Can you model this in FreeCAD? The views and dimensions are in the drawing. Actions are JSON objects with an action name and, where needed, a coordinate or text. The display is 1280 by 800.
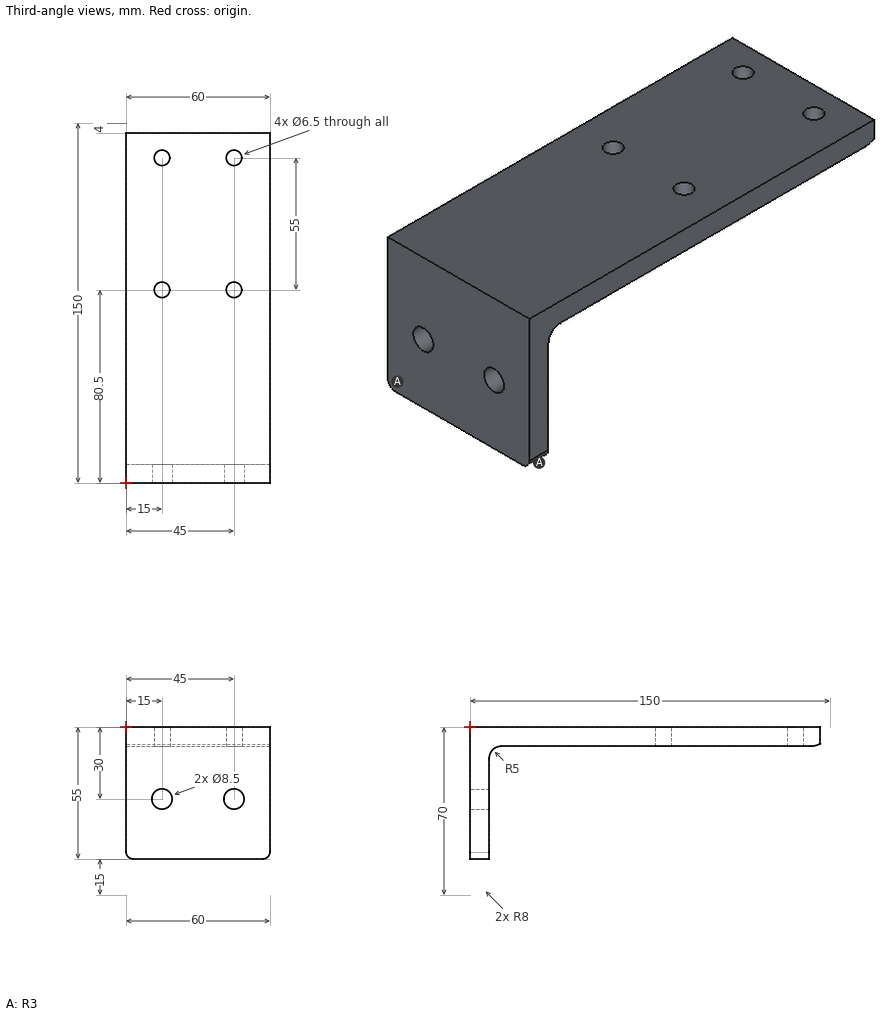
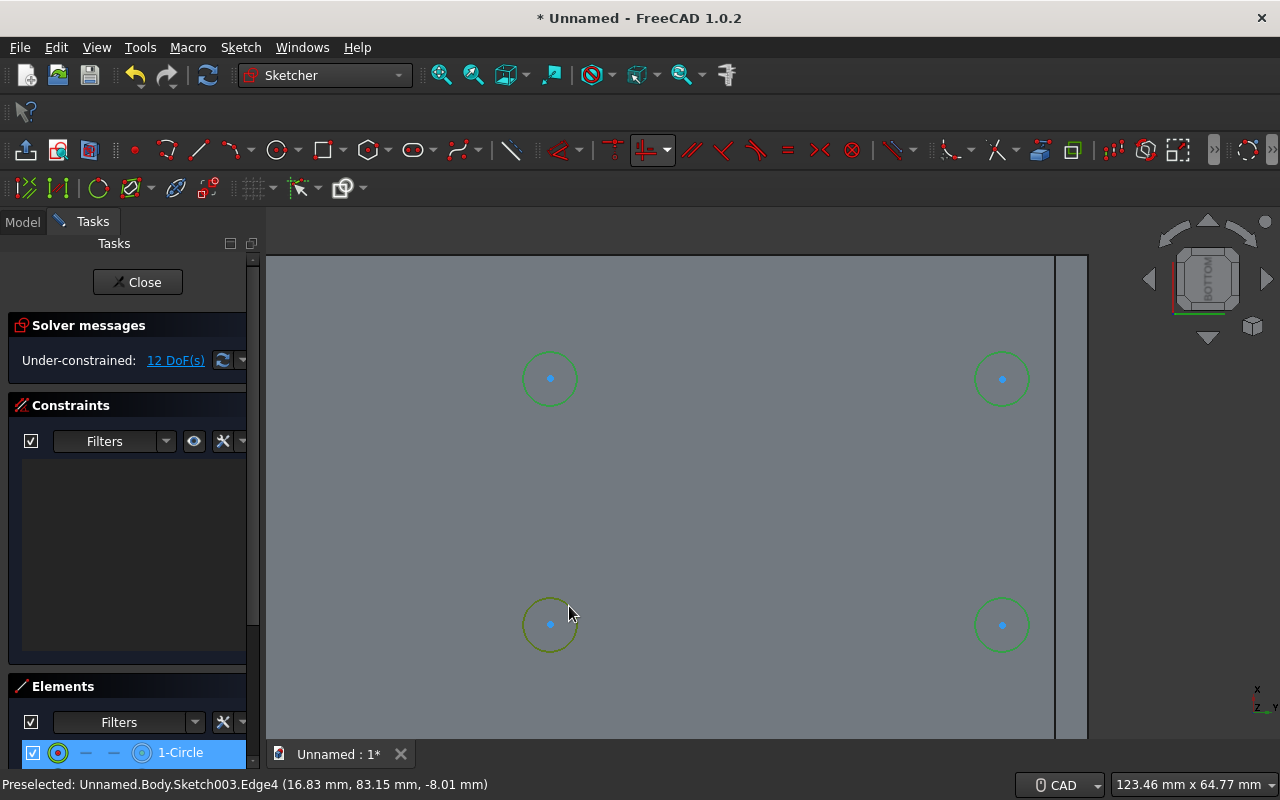
{"action": "key", "text": "e"}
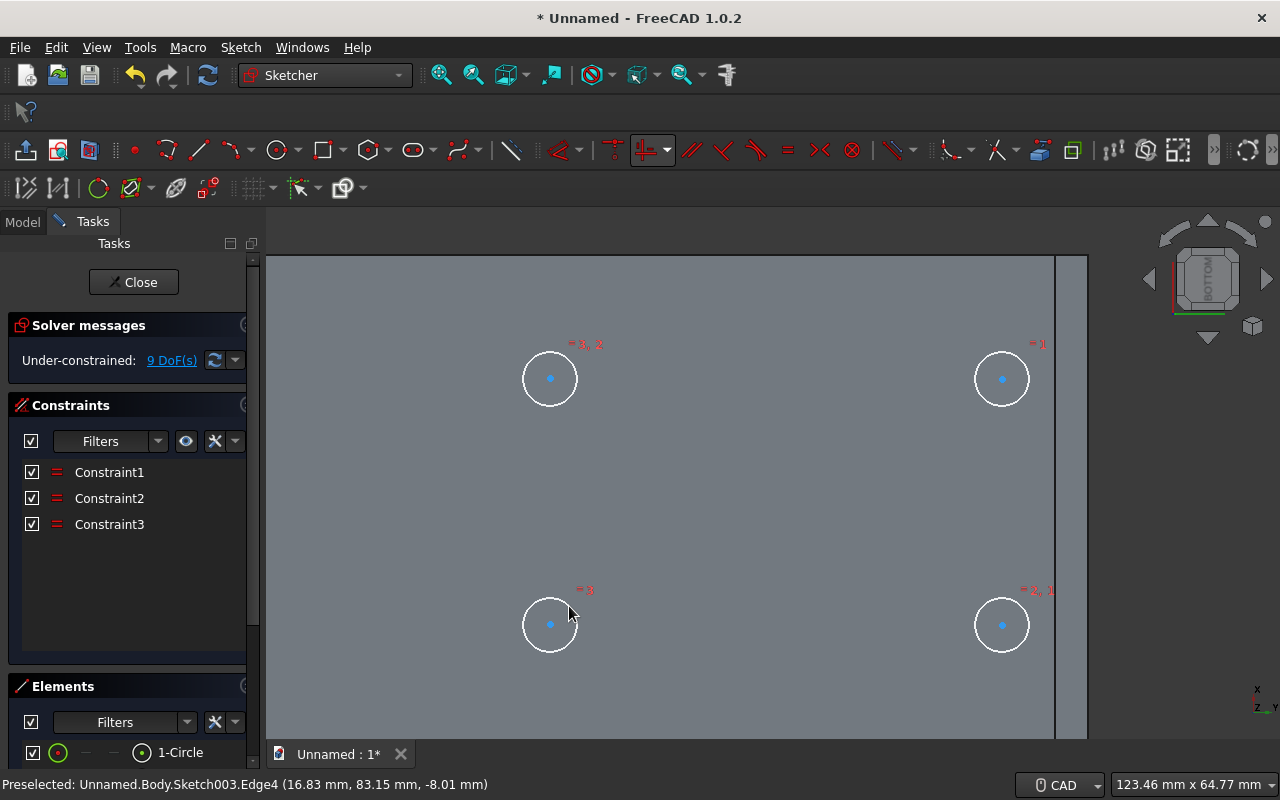
{"action": "left_click", "coordinate": [558, 150]}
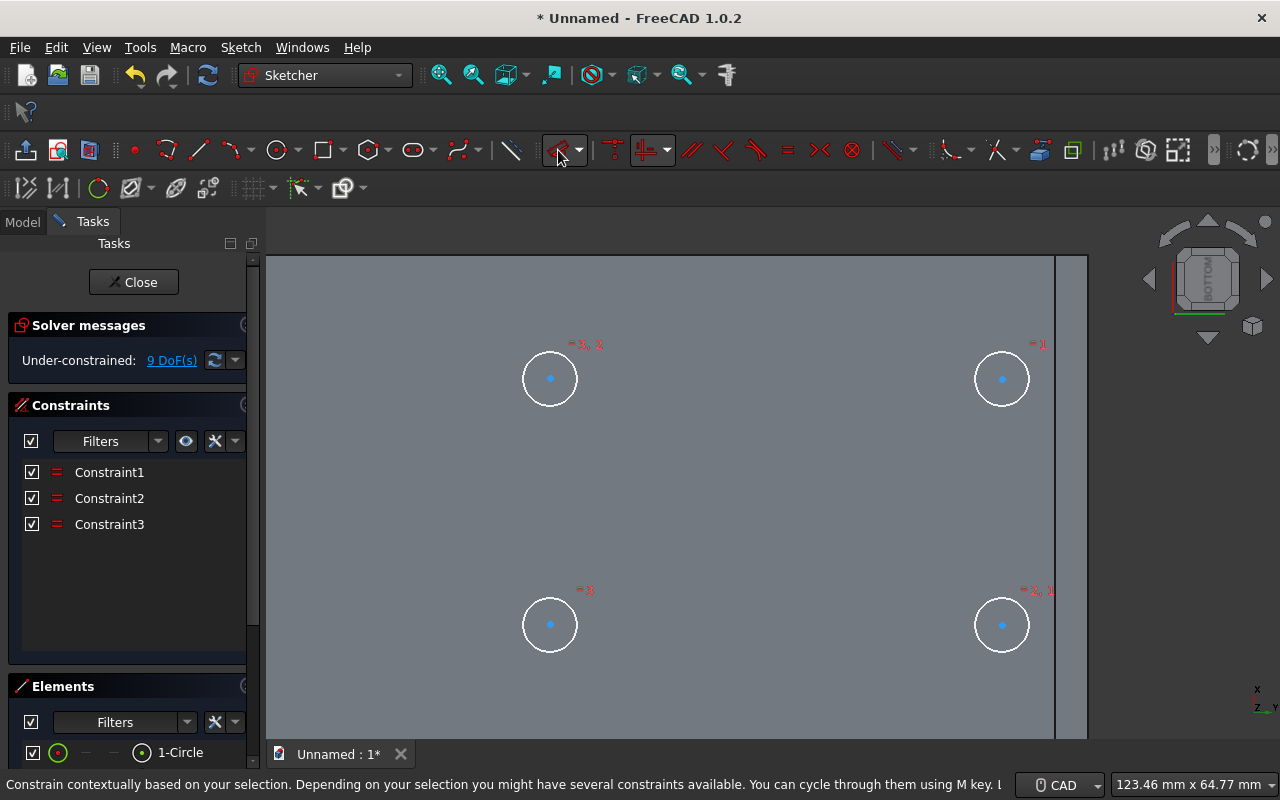
{"action": "left_click", "coordinate": [1021, 360]}
{"action": "left_click", "coordinate": [1044, 337]}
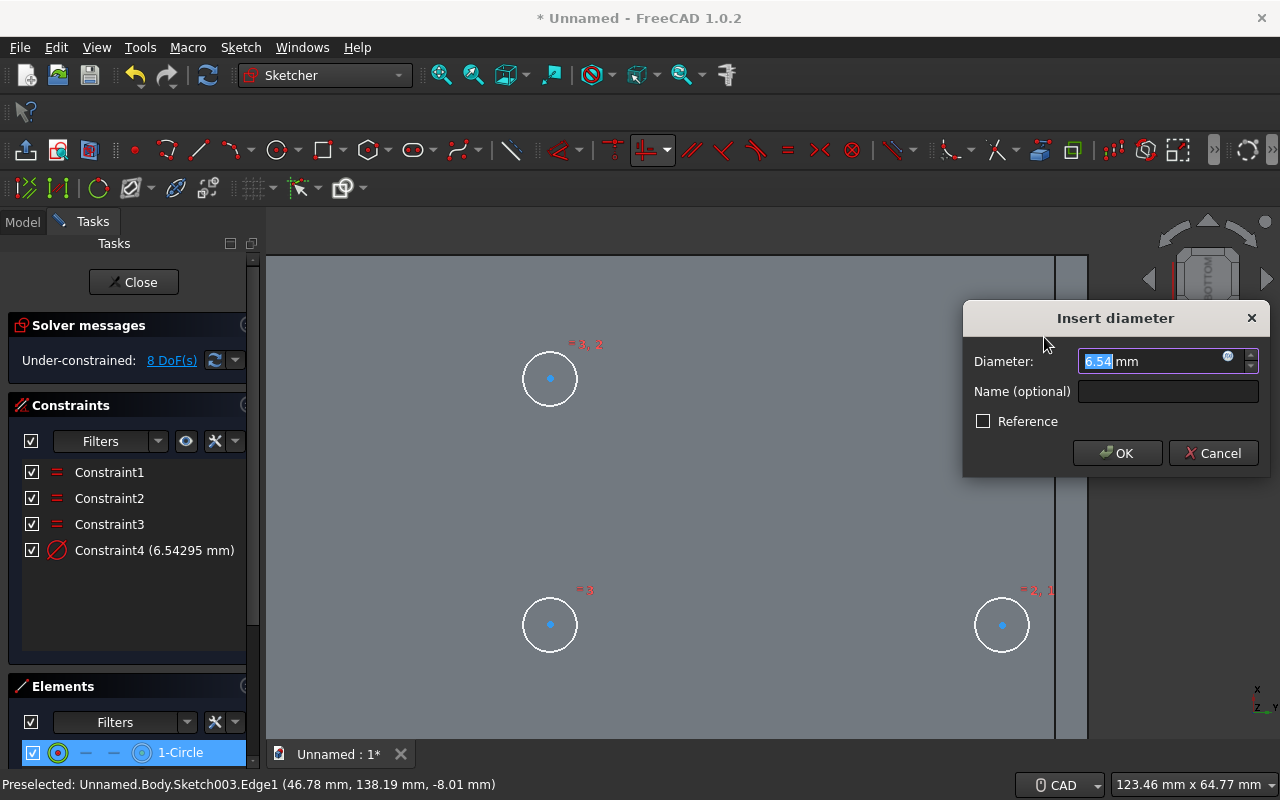
{"action": "type", "text": "6.5"}
{"action": "key", "text": "Return"}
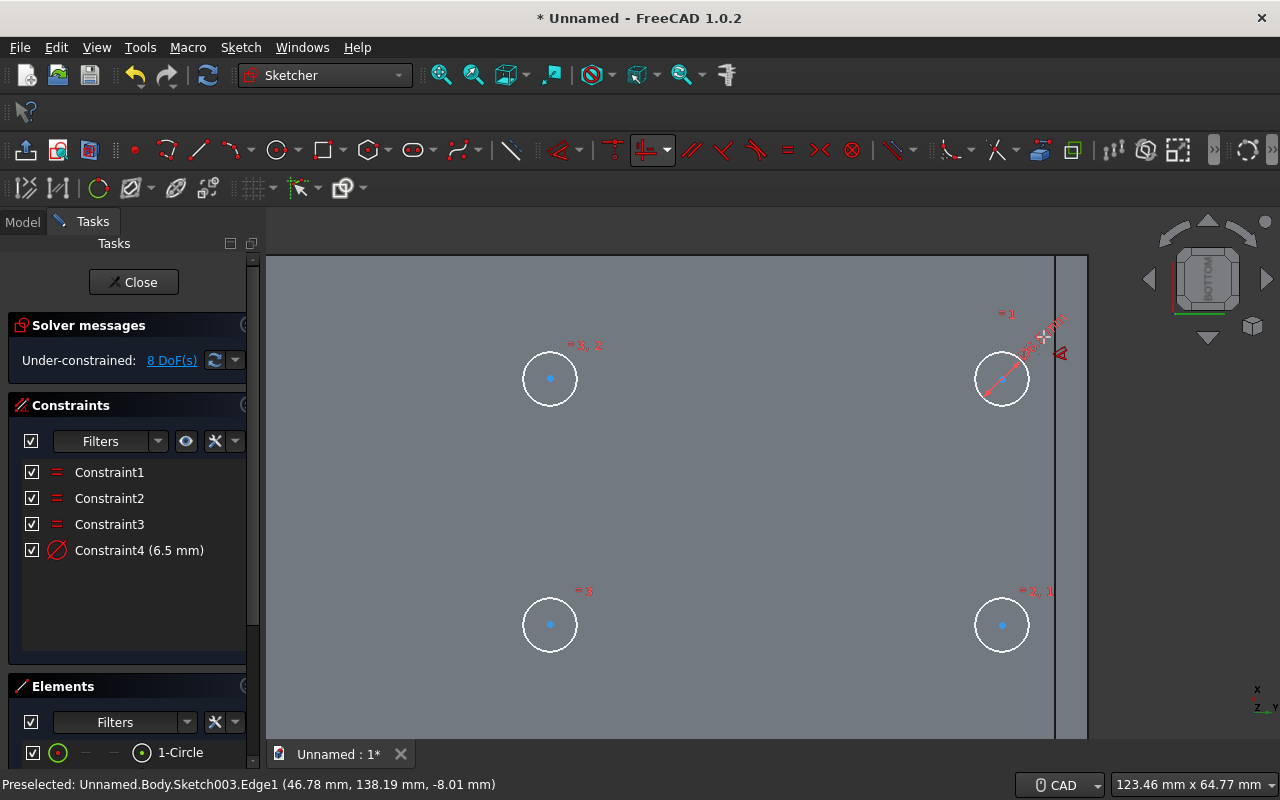
{"action": "left_click", "coordinate": [1002, 379]}
{"action": "left_click", "coordinate": [1036, 545]}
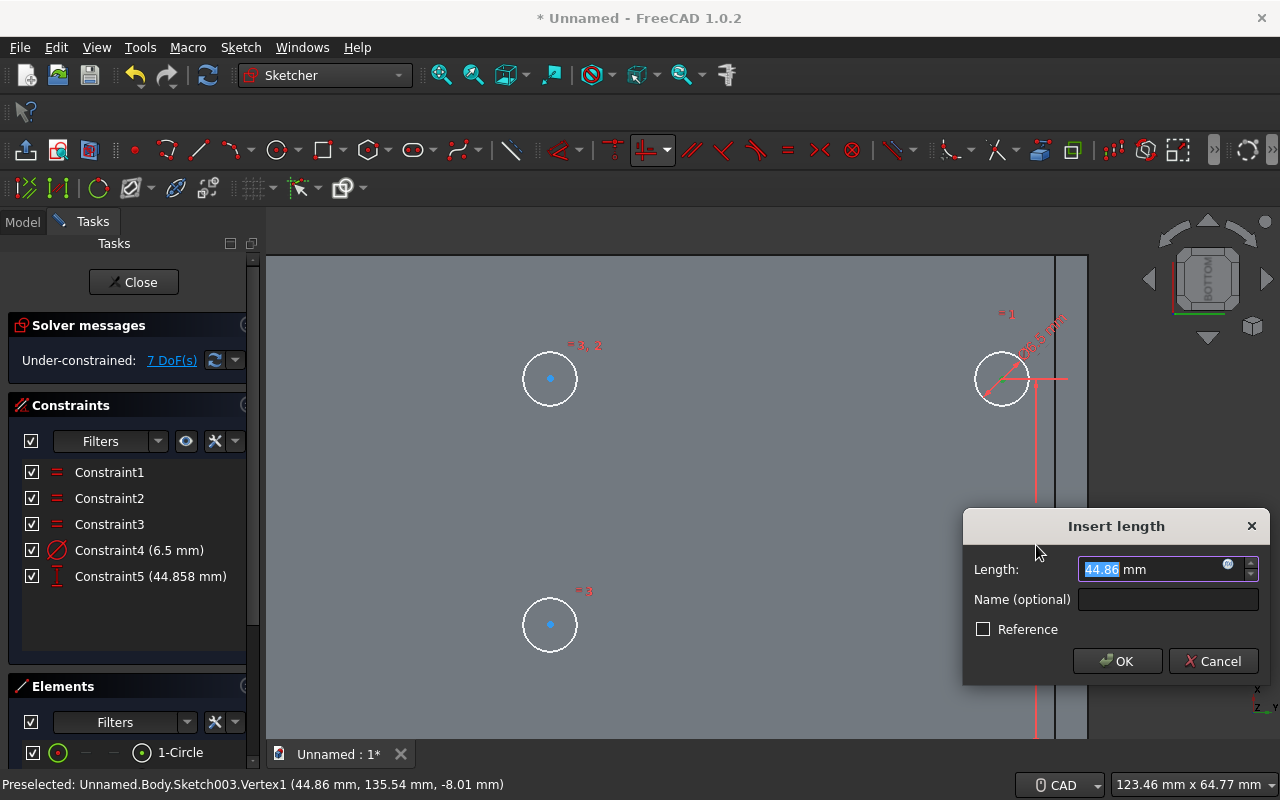
{"action": "type", "text": "45"}
{"action": "key", "text": "Return"}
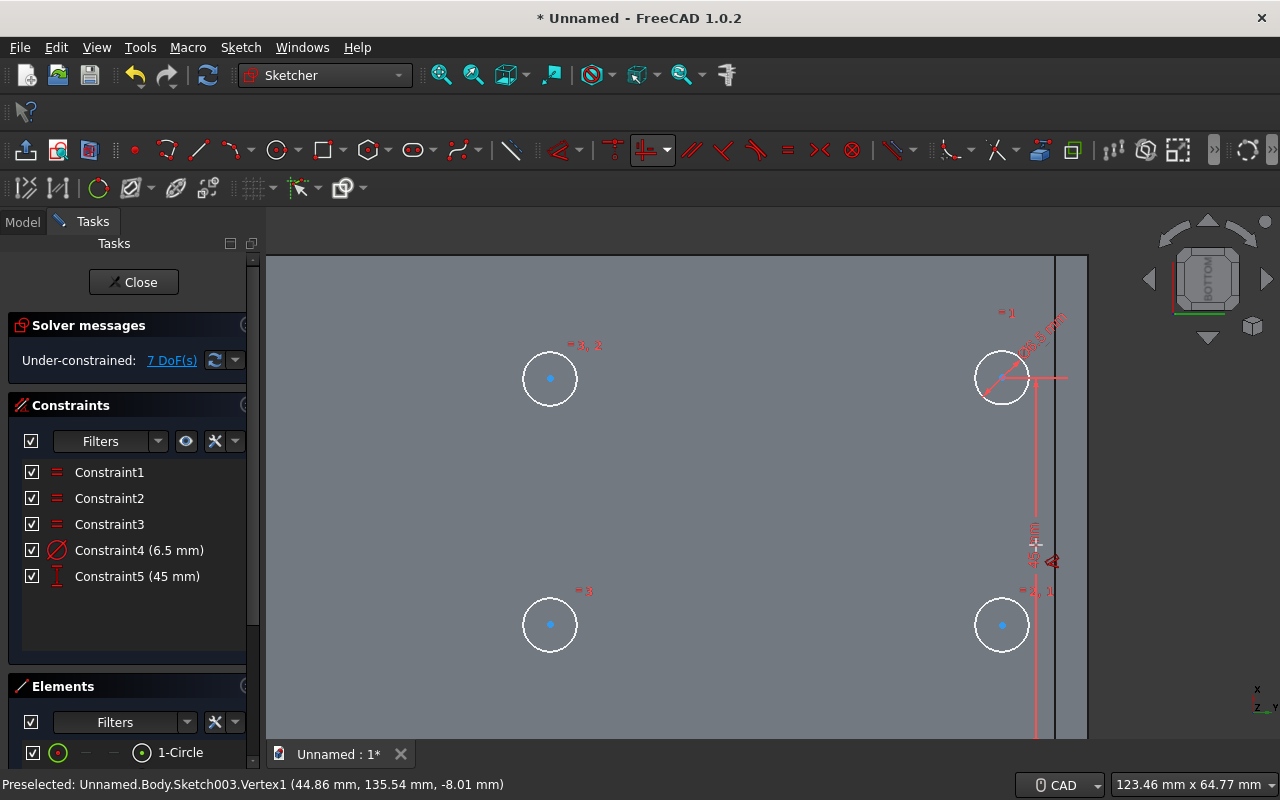
{"action": "left_click", "coordinate": [1002, 625]}
{"action": "left_click", "coordinate": [1036, 668]}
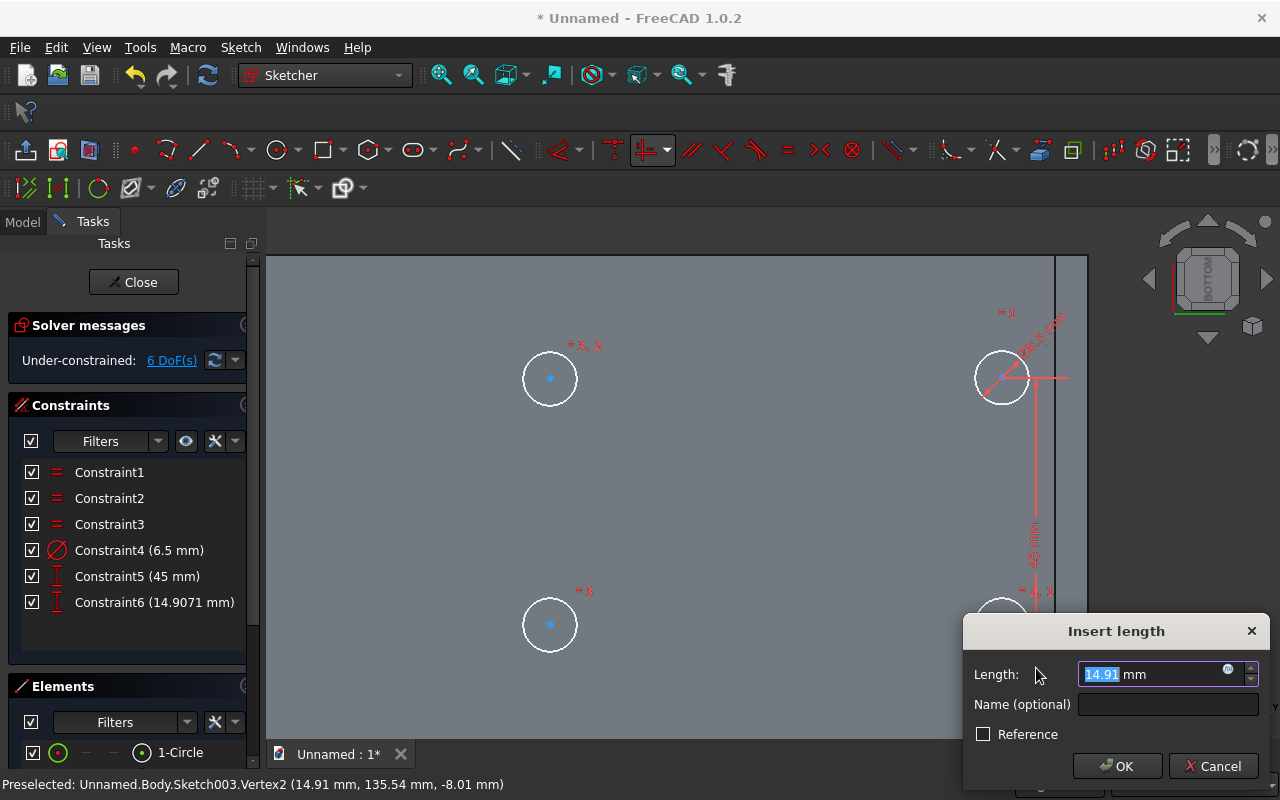
{"action": "type", "text": "15"}
{"action": "key", "text": "Return"}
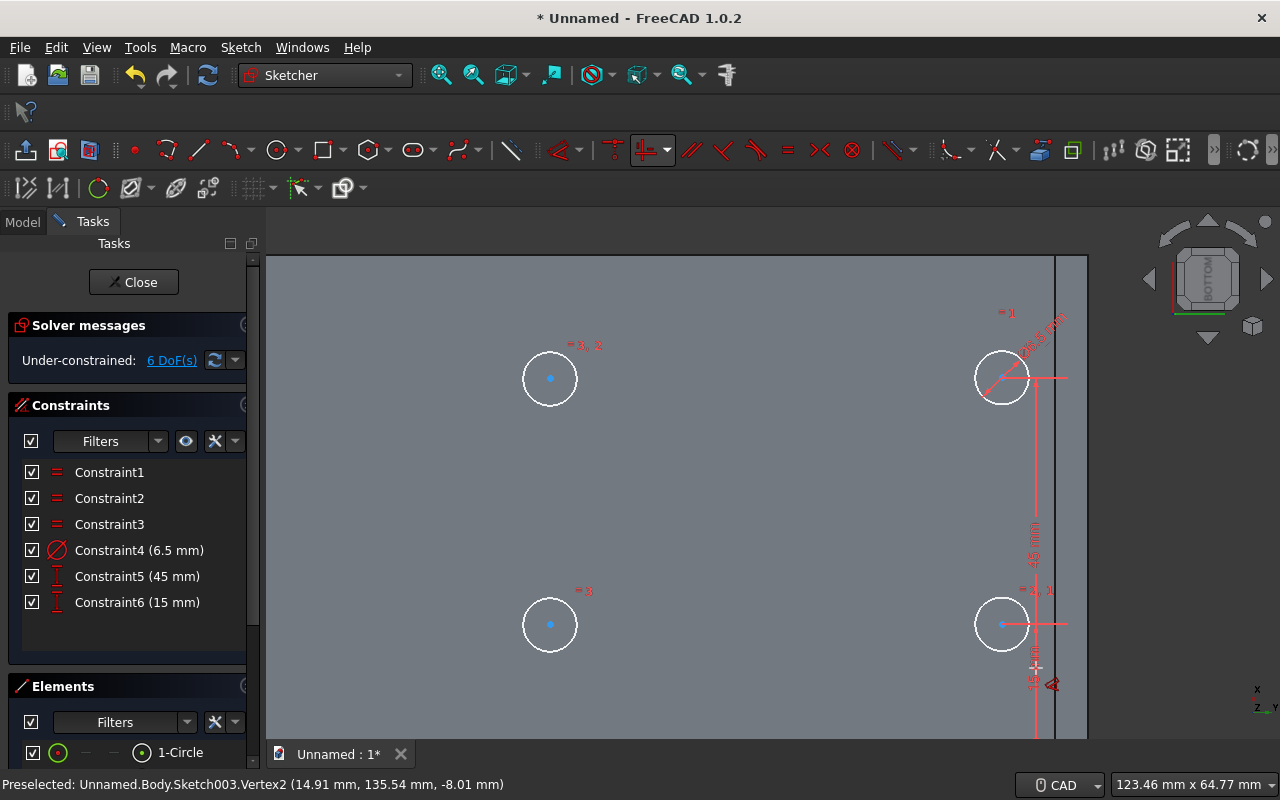
{"action": "left_click", "coordinate": [550, 379]}
{"action": "left_click", "coordinate": [584, 545]}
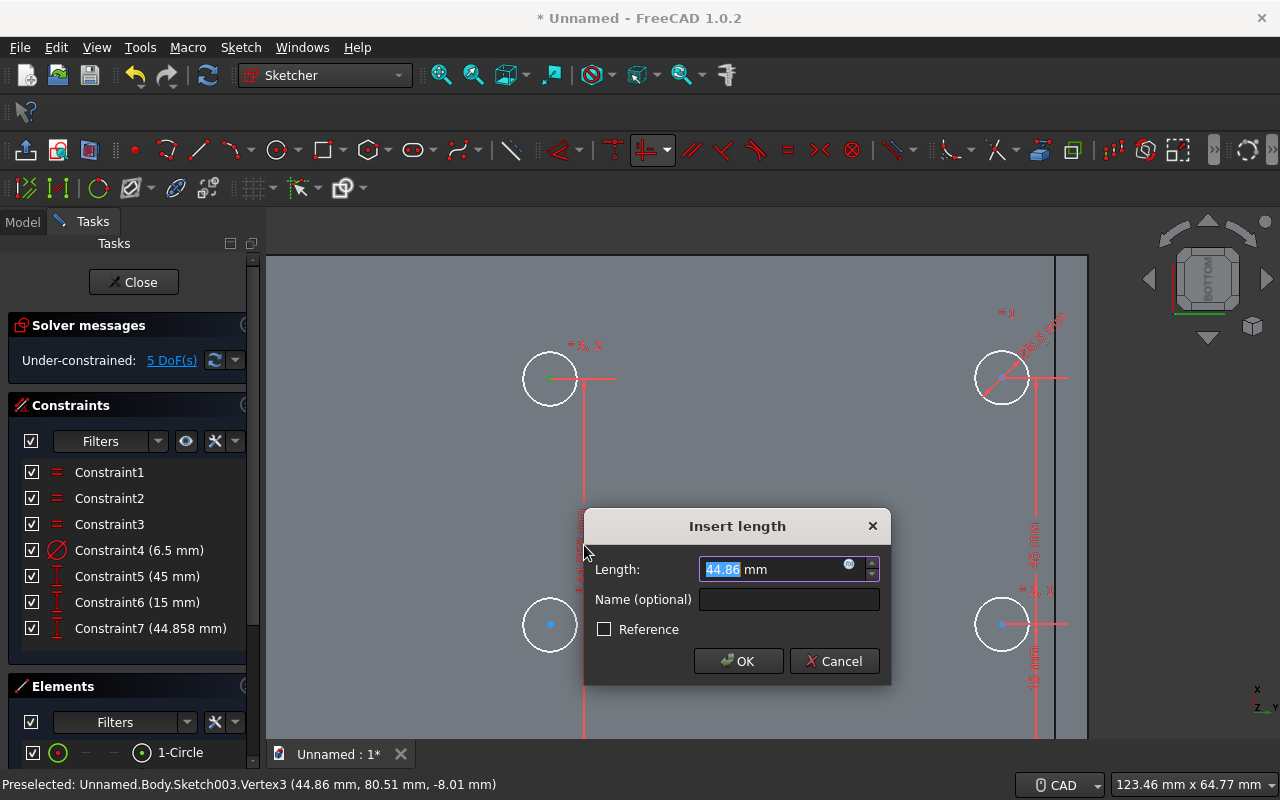
{"action": "type", "text": "45"}
{"action": "key", "text": "Return"}